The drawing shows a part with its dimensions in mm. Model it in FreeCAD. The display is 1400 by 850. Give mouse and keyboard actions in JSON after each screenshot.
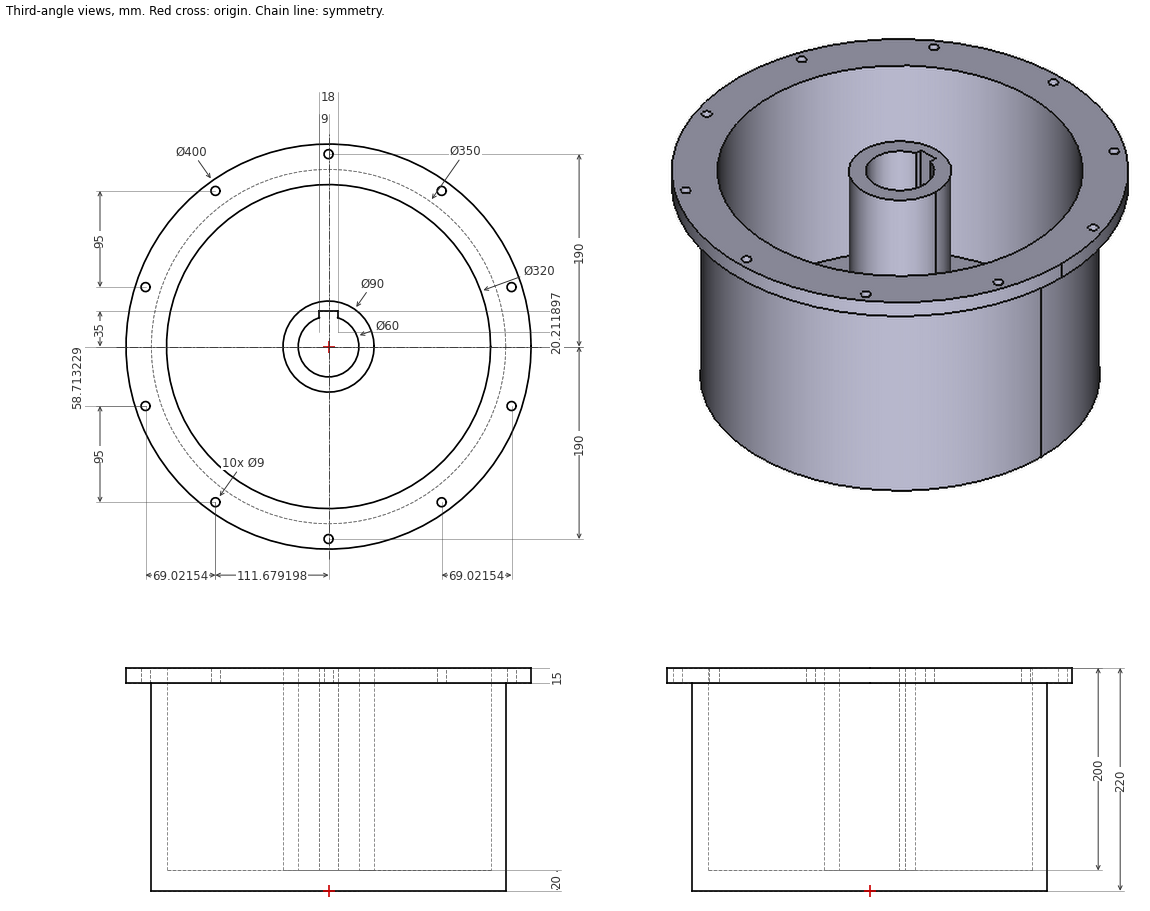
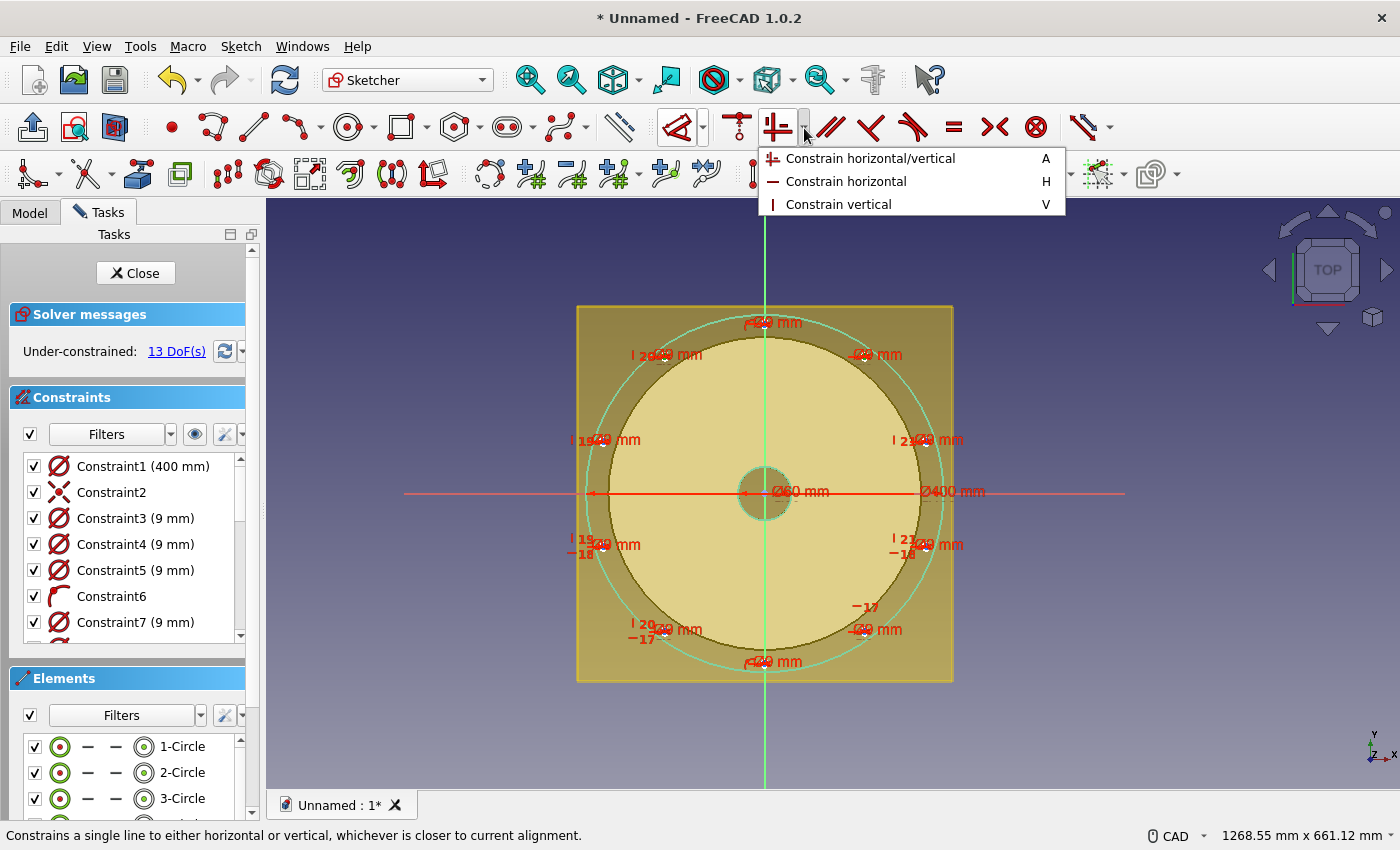
{"action": "left_click", "coordinate": [912, 182]}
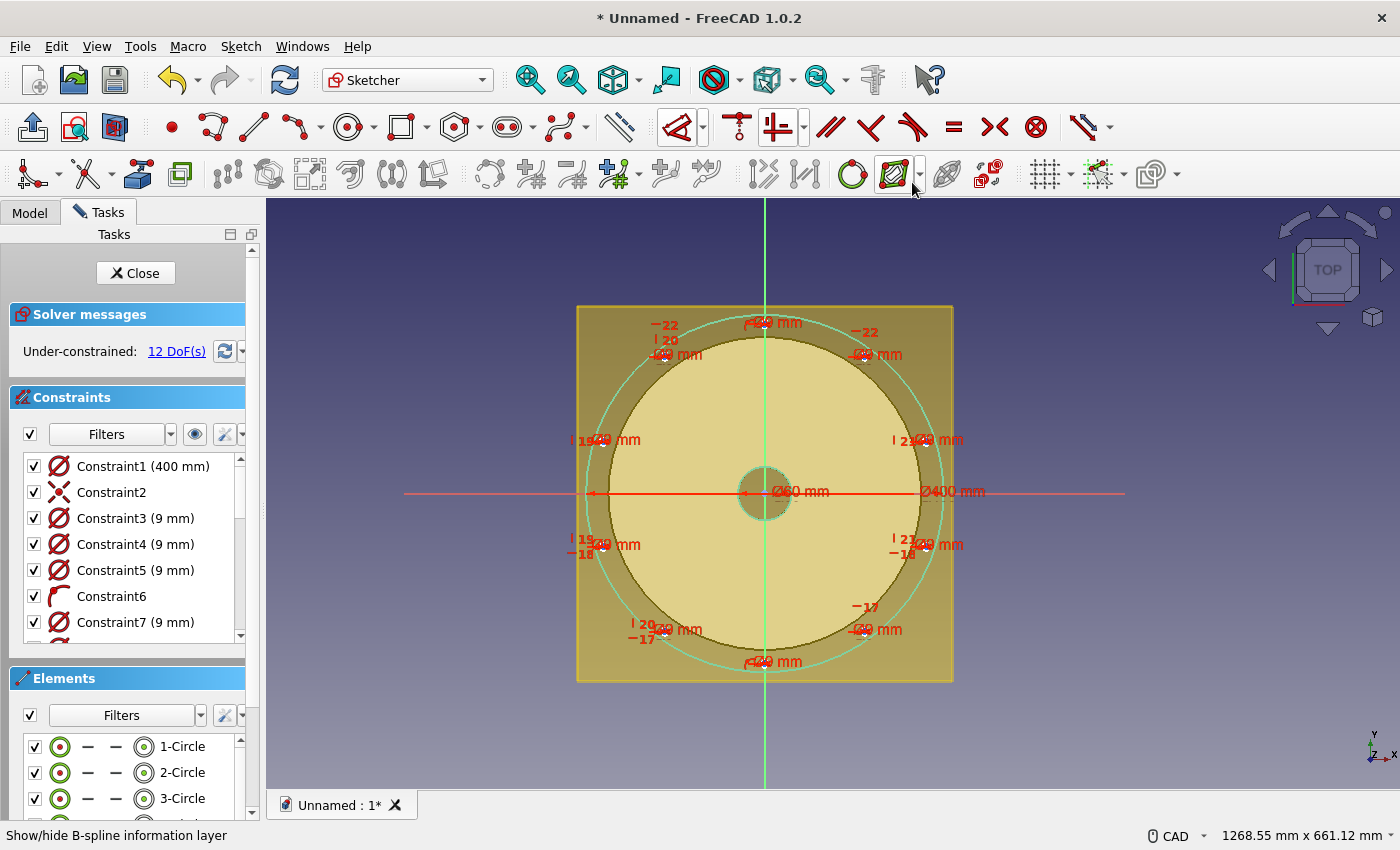
{"action": "left_click", "coordinate": [603, 442]}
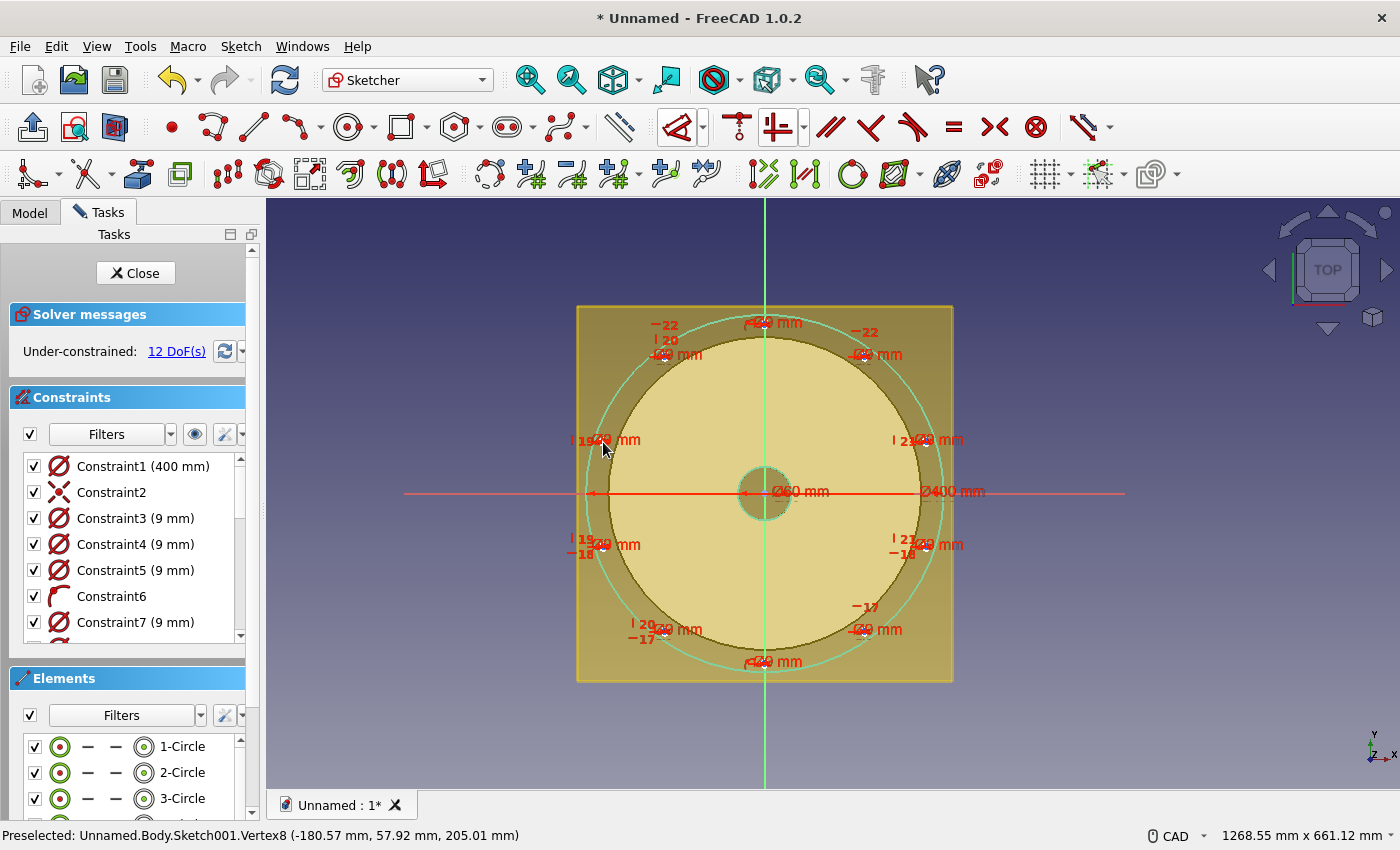
{"action": "left_click", "coordinate": [926, 442]}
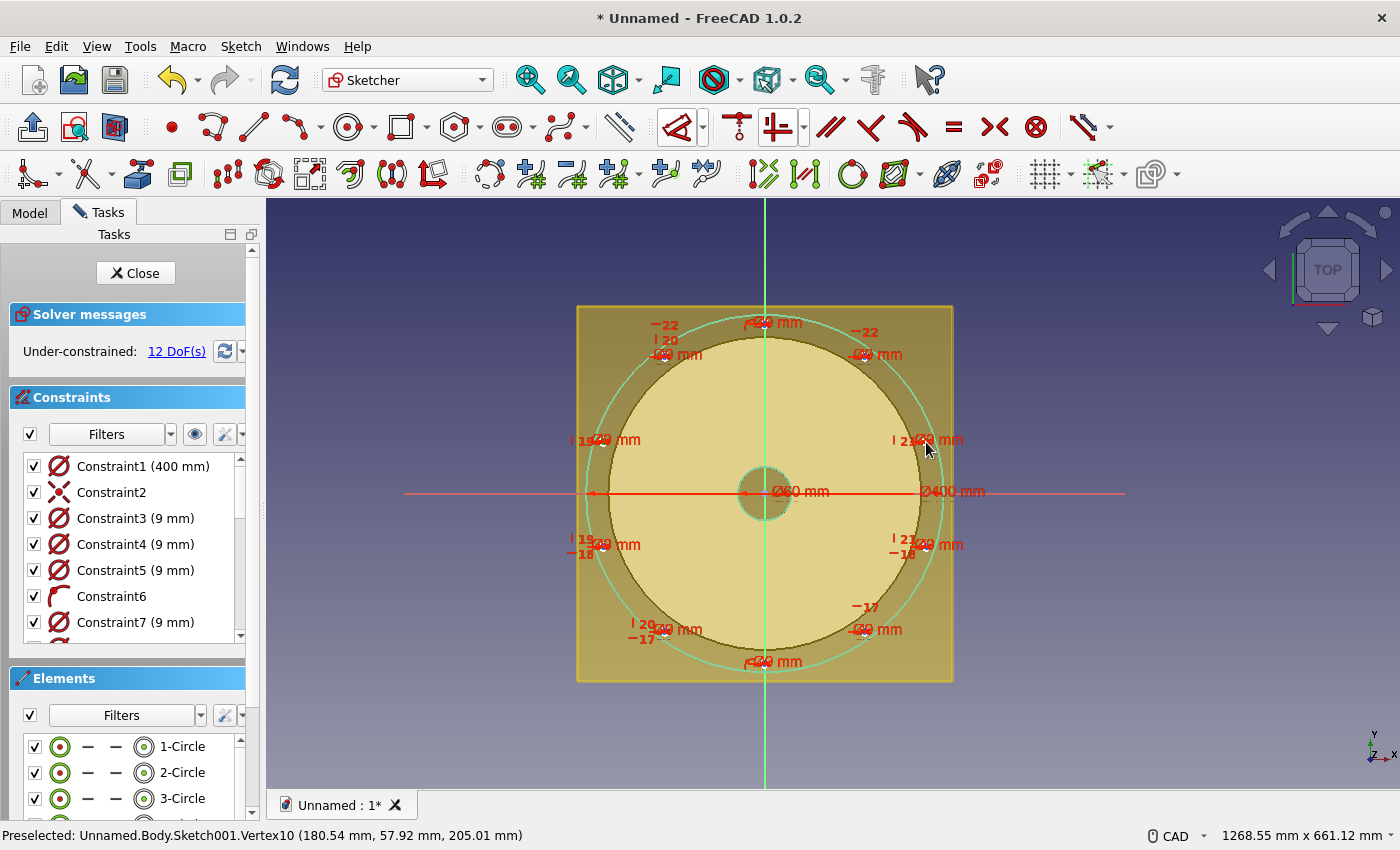
{"action": "left_click", "coordinate": [765, 723]}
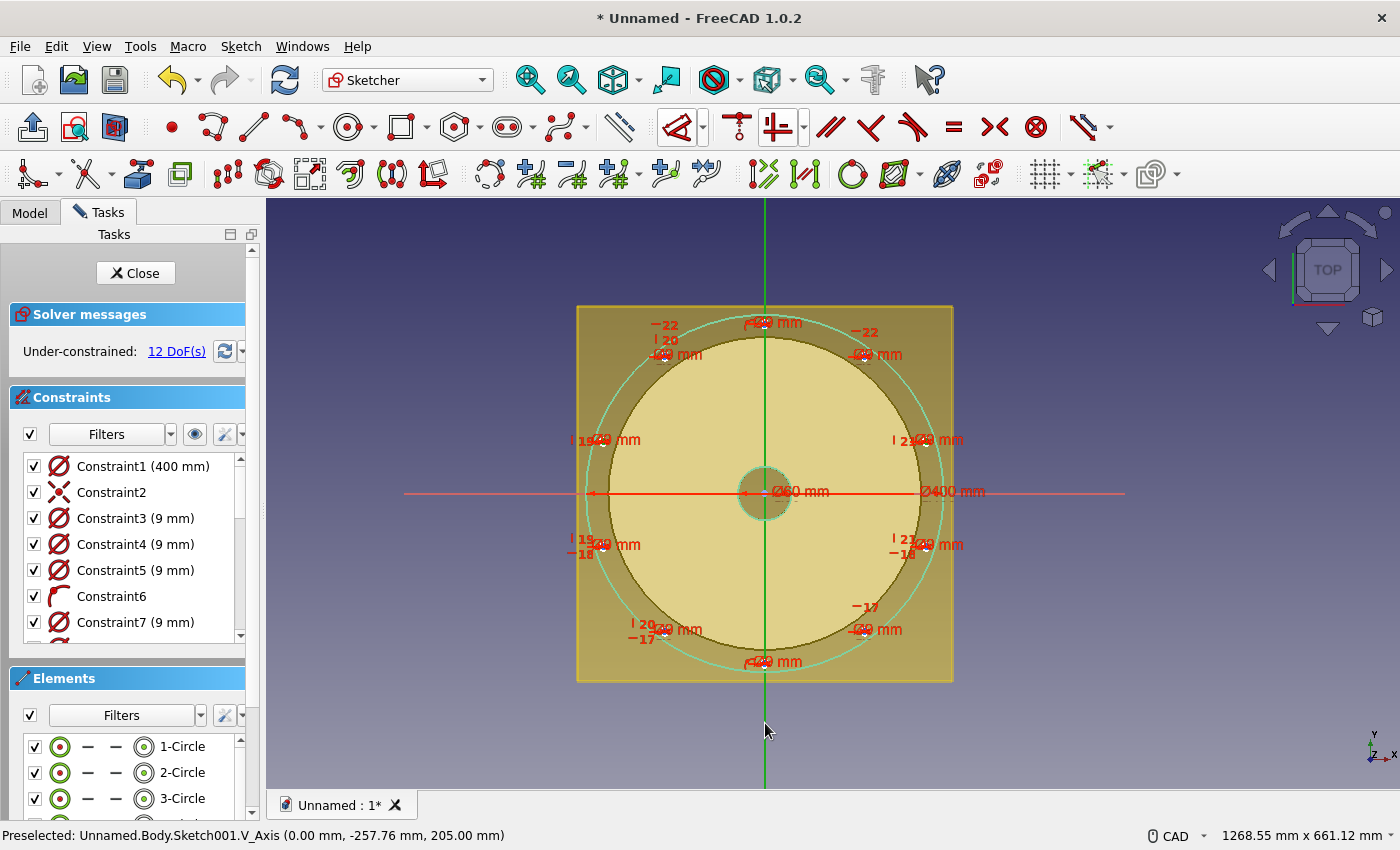
{"action": "left_click", "coordinate": [995, 128]}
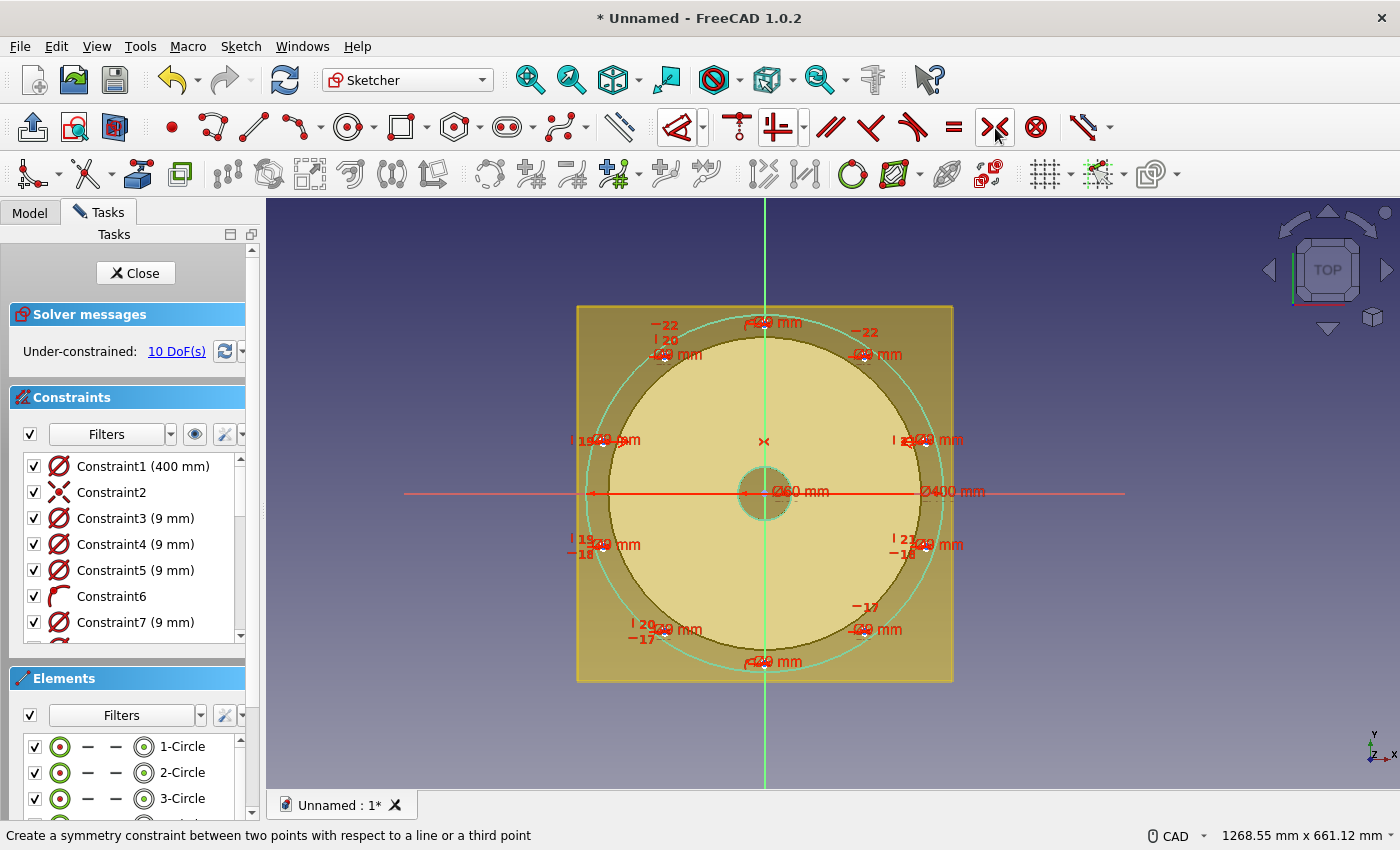
{"action": "left_click", "coordinate": [865, 632]}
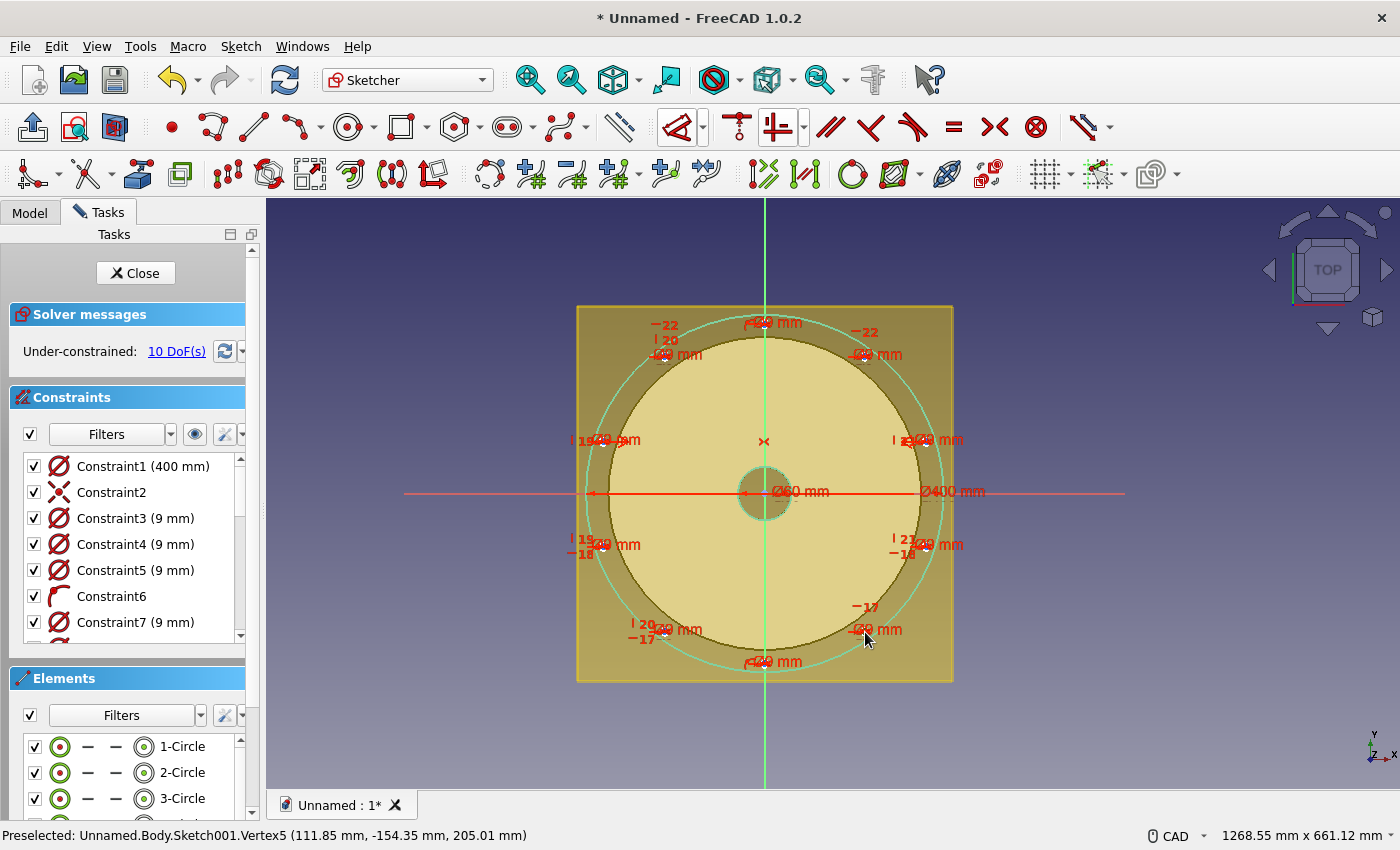
{"action": "left_click", "coordinate": [865, 357]}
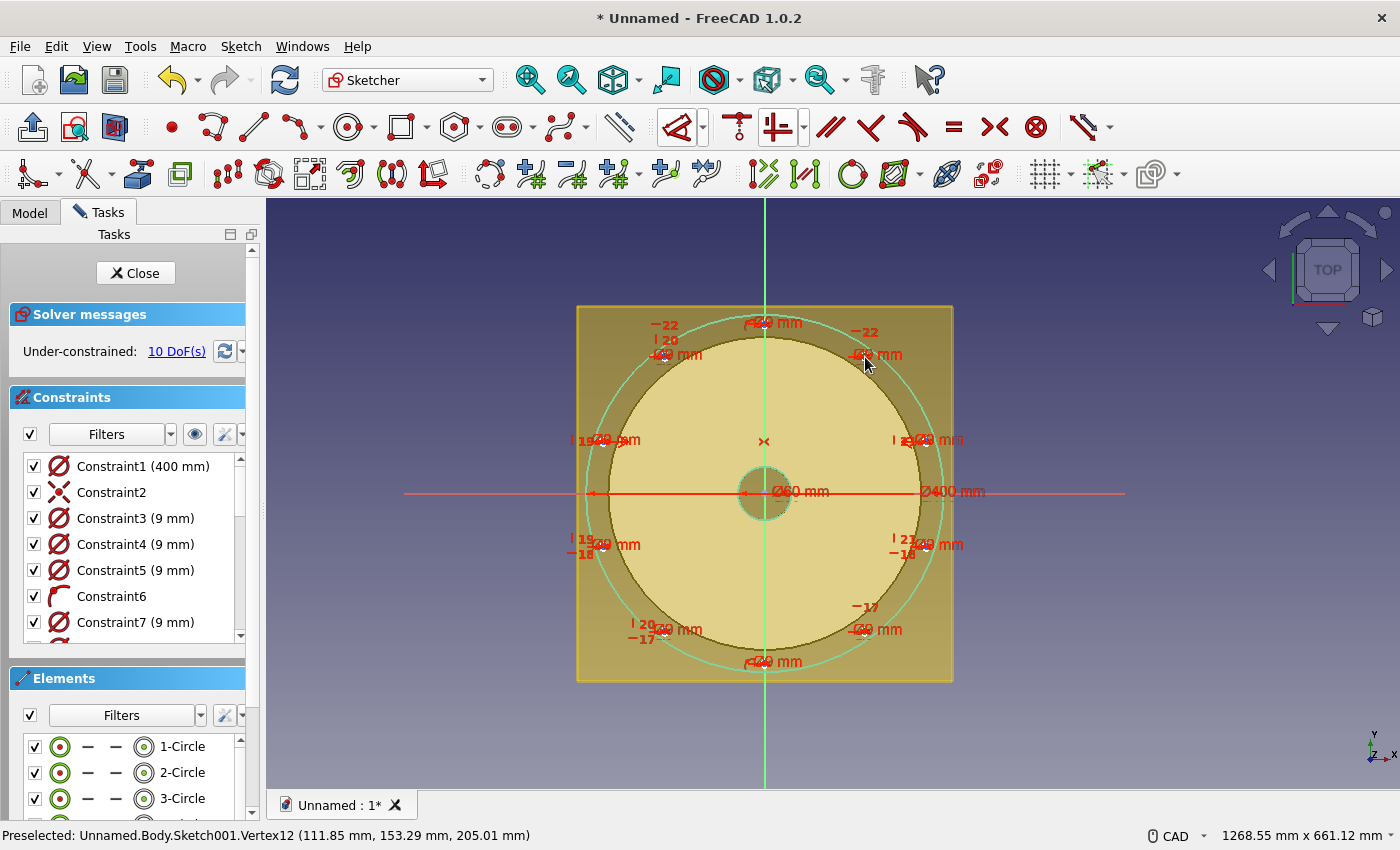
{"action": "left_click", "coordinate": [428, 494]}